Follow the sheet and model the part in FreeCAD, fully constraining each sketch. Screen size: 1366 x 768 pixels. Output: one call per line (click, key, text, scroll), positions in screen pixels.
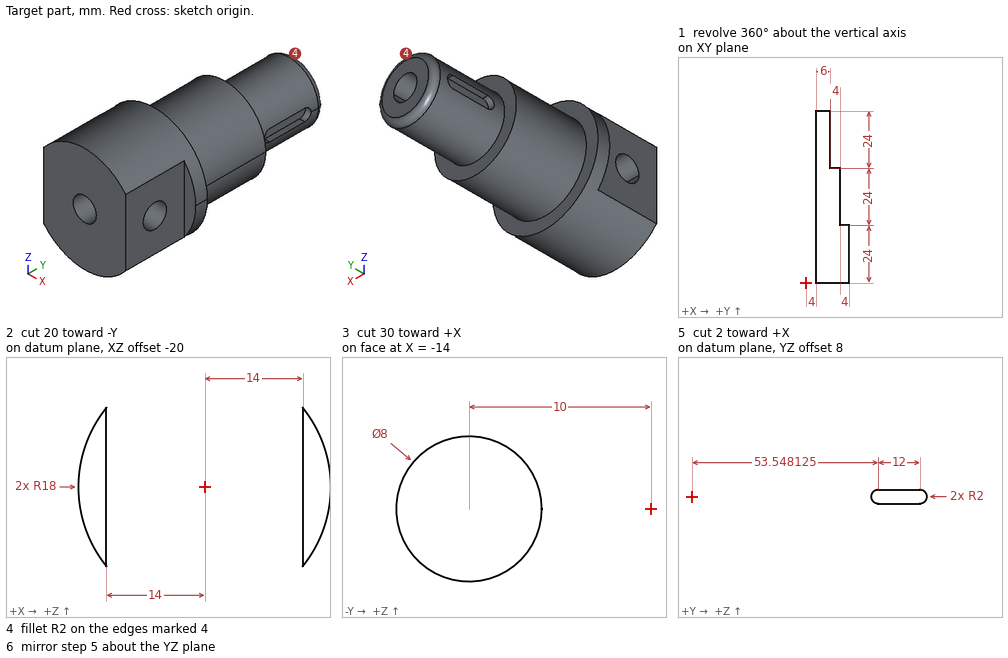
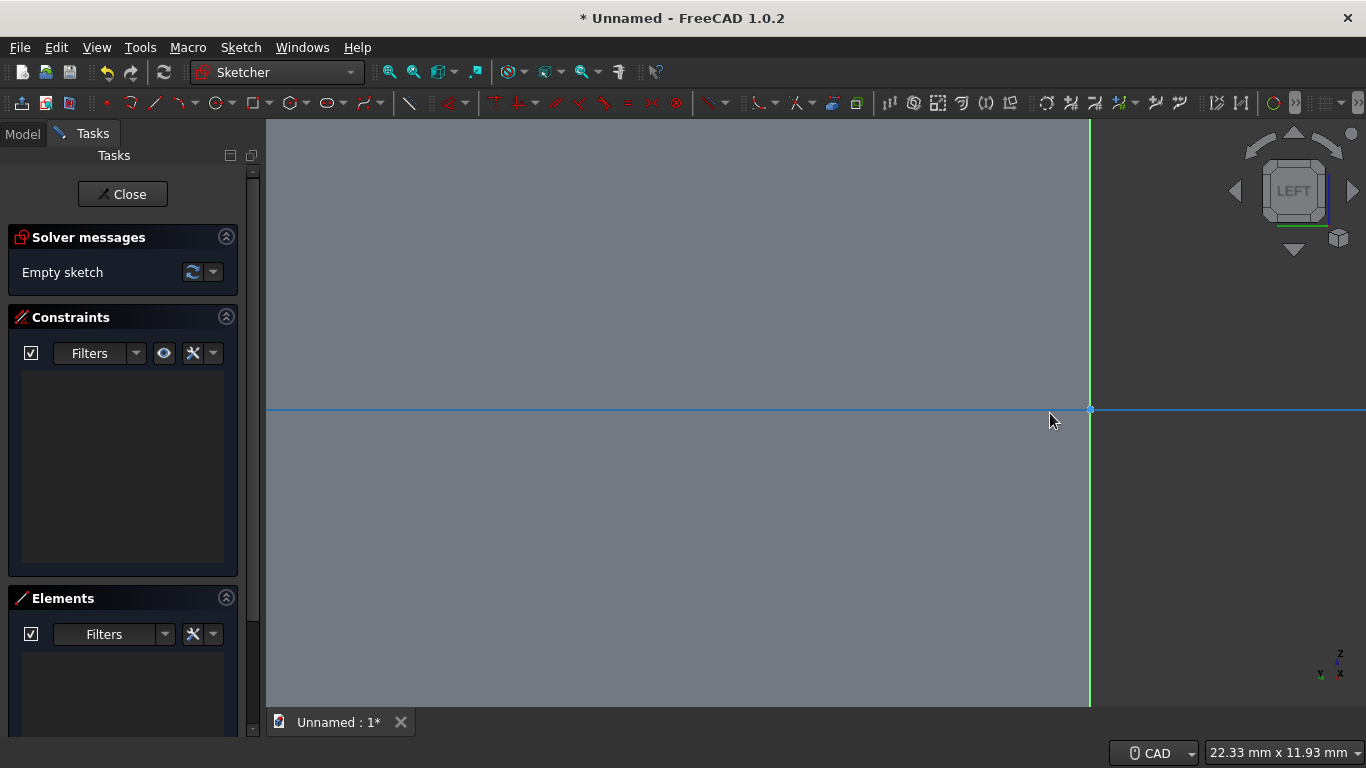
click(216, 104)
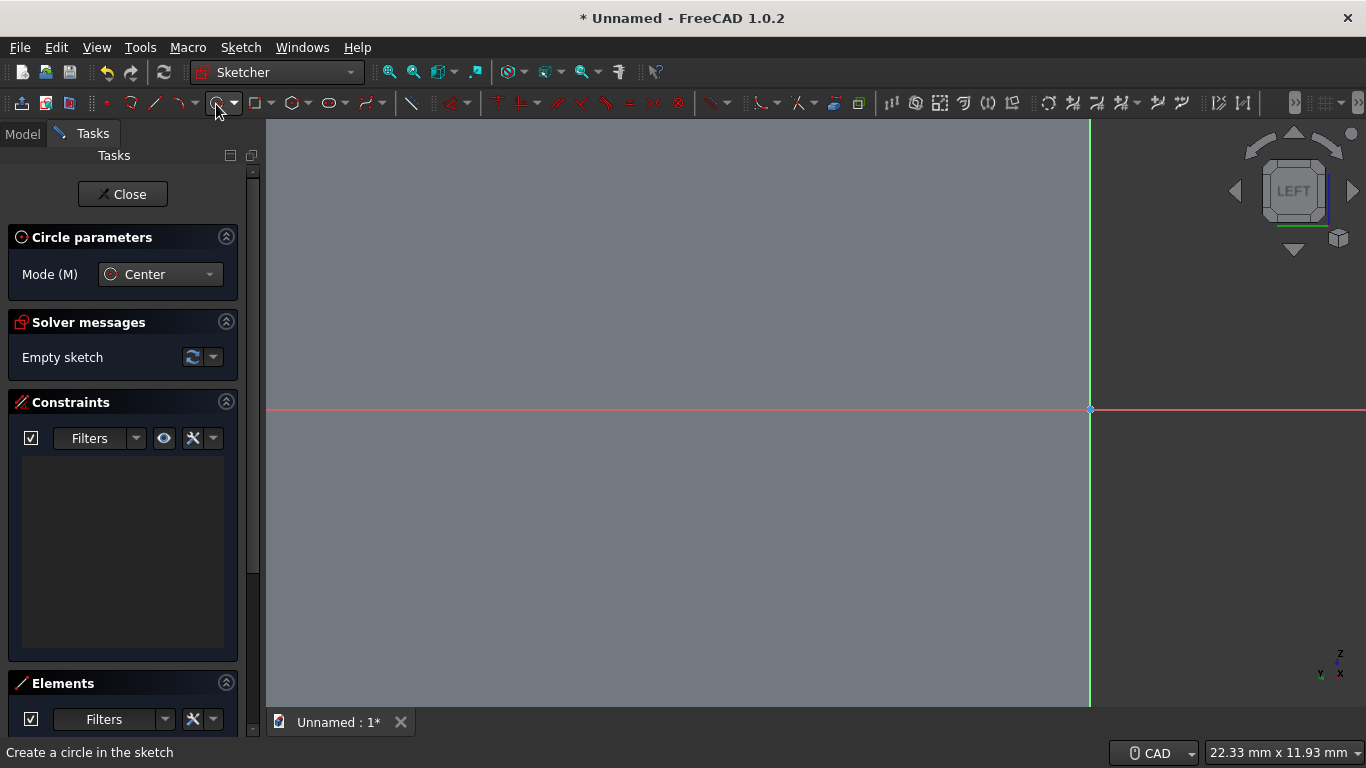
click(597, 410)
click(737, 270)
key(Escape)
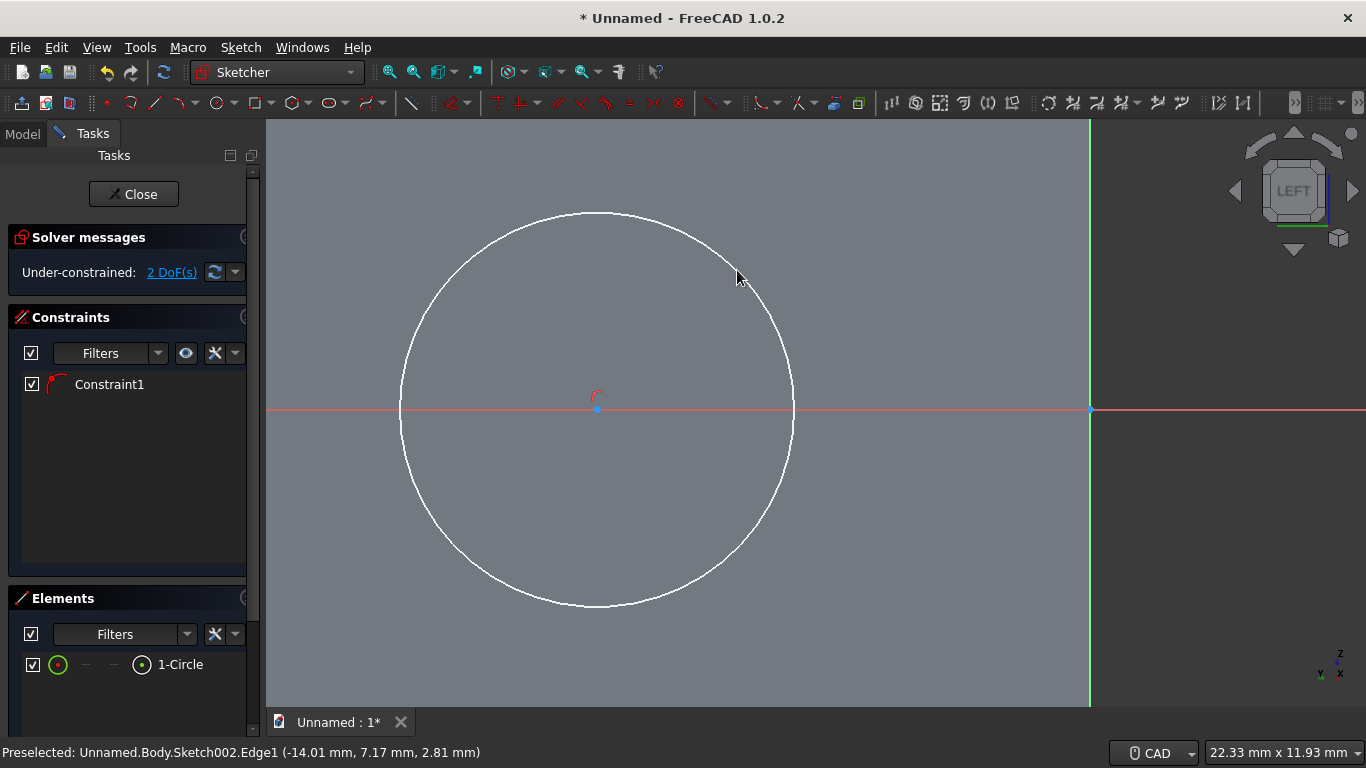
click(450, 104)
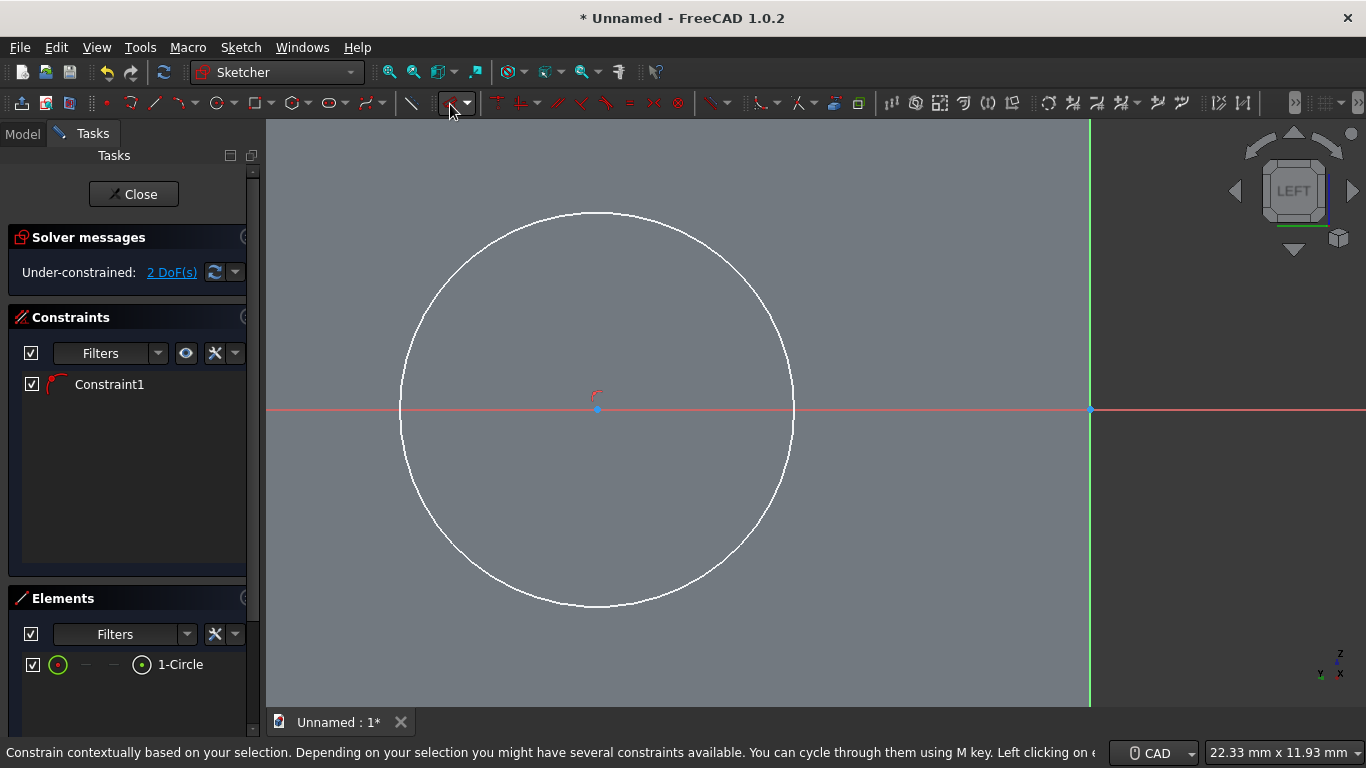
click(736, 270)
click(759, 247)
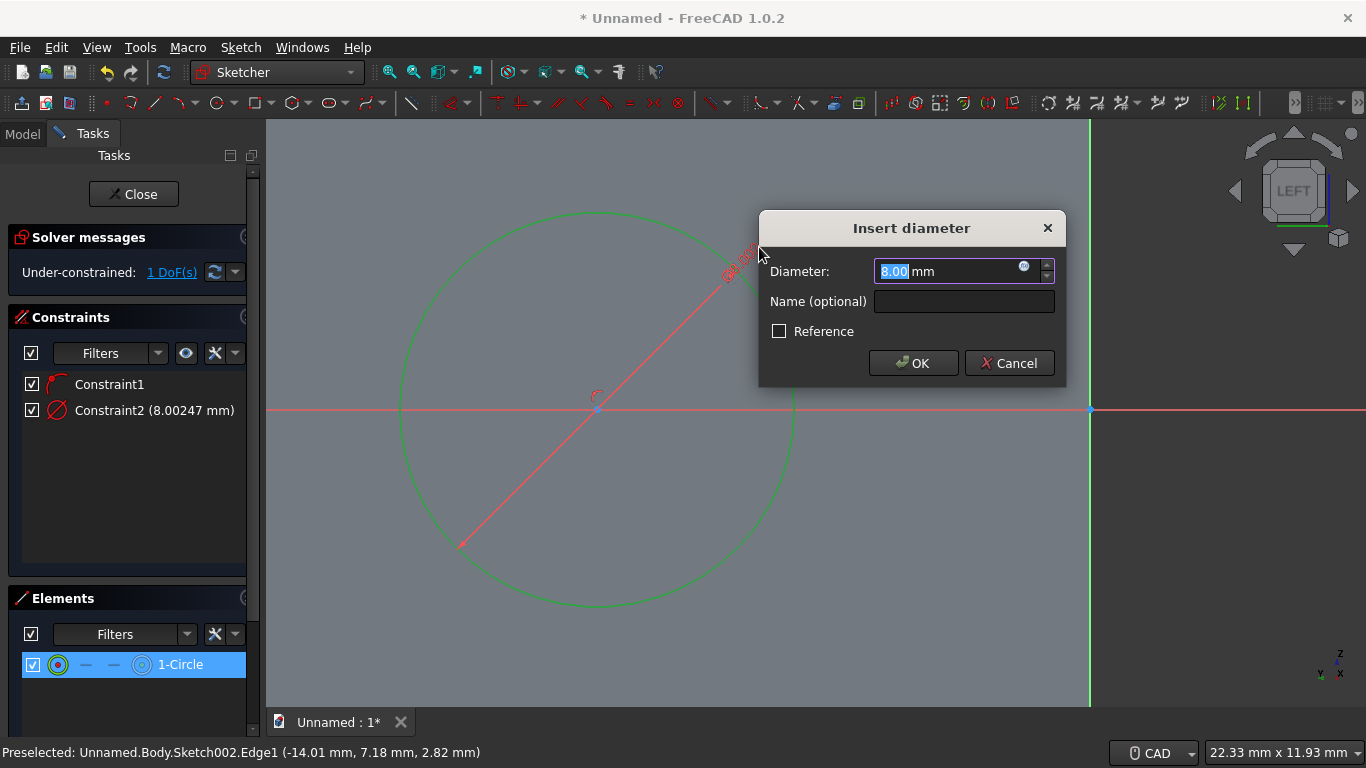
text(8)
key(Return)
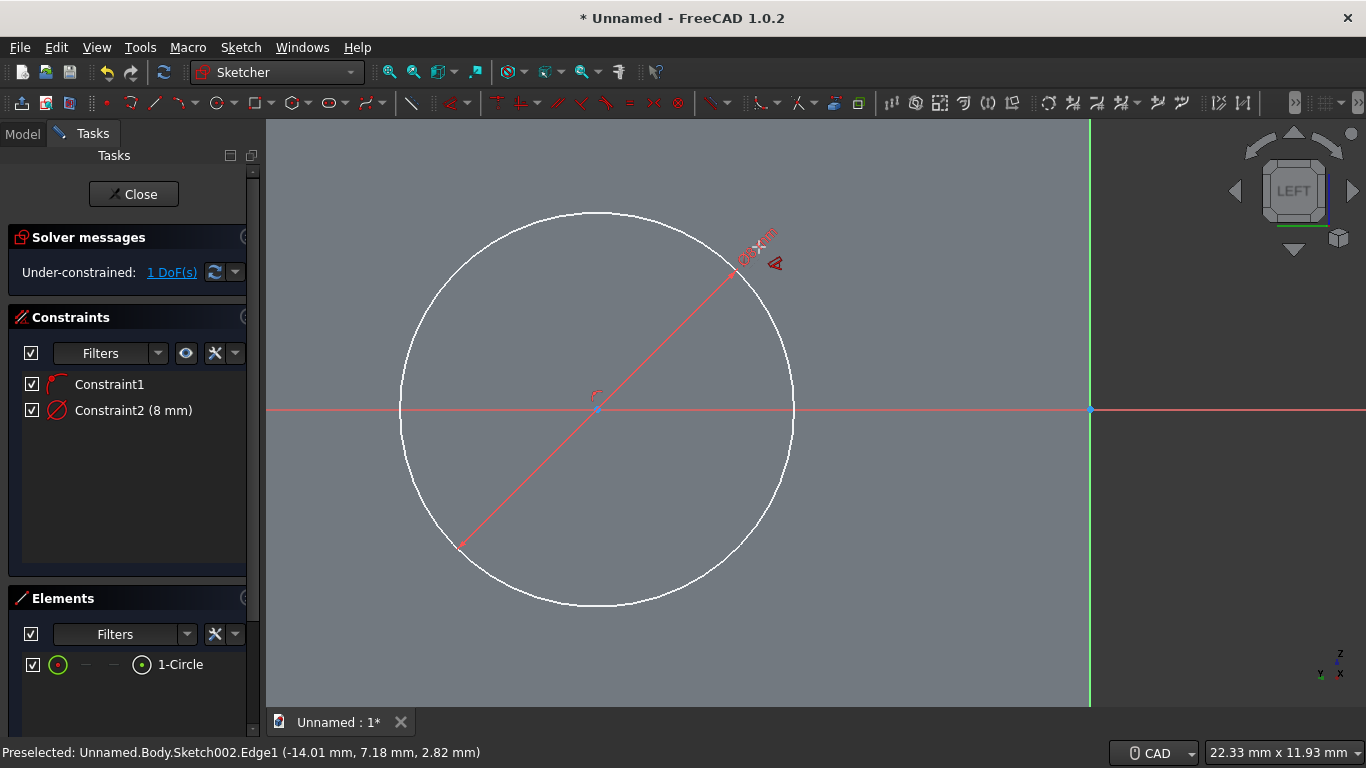
click(597, 410)
click(844, 444)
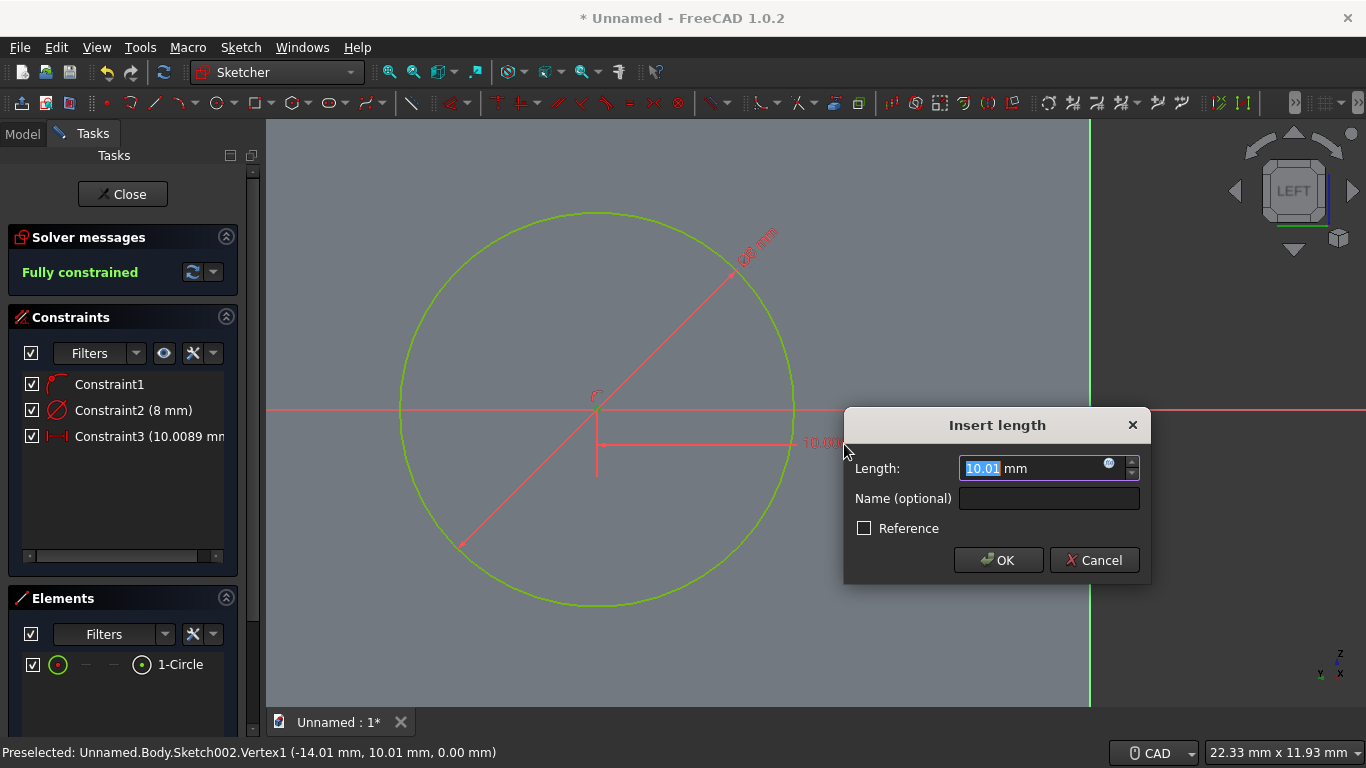
text(10)
key(Return)
key(Escape)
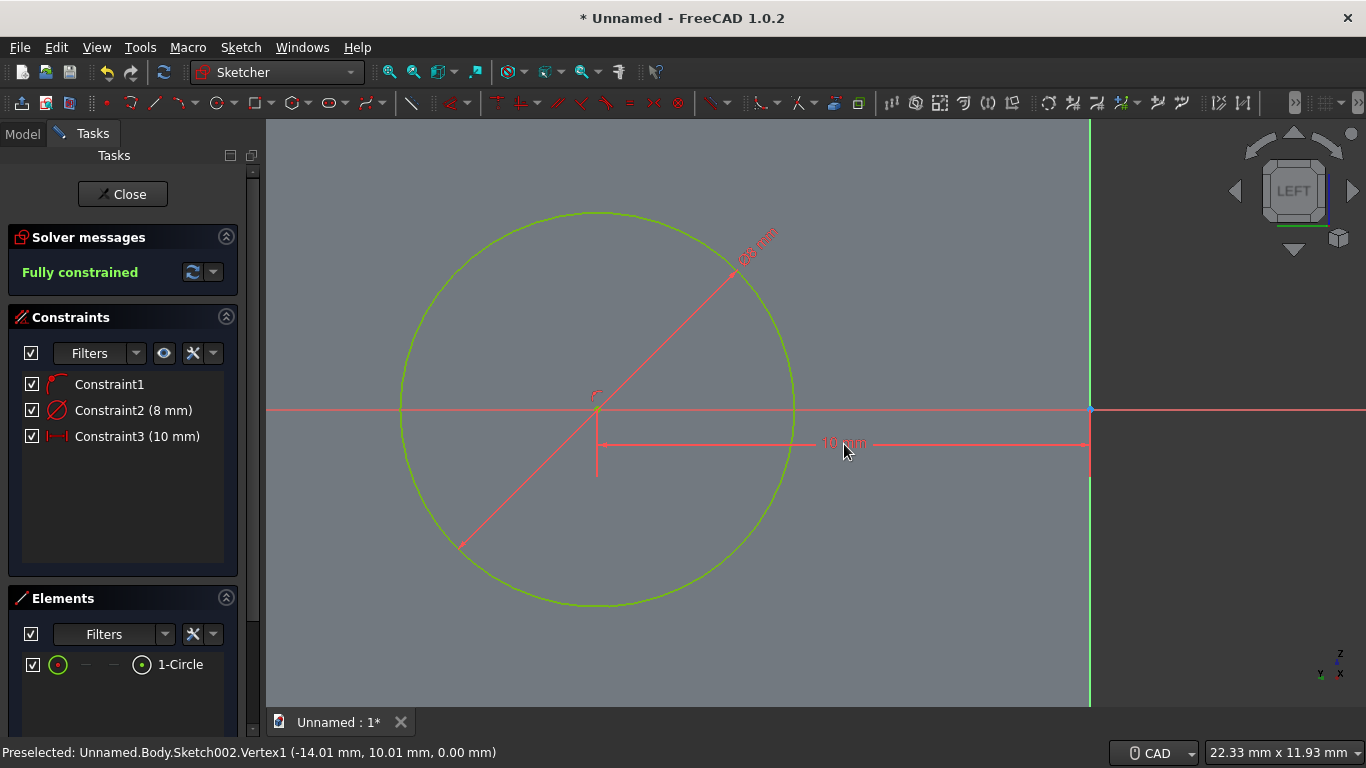
click(123, 194)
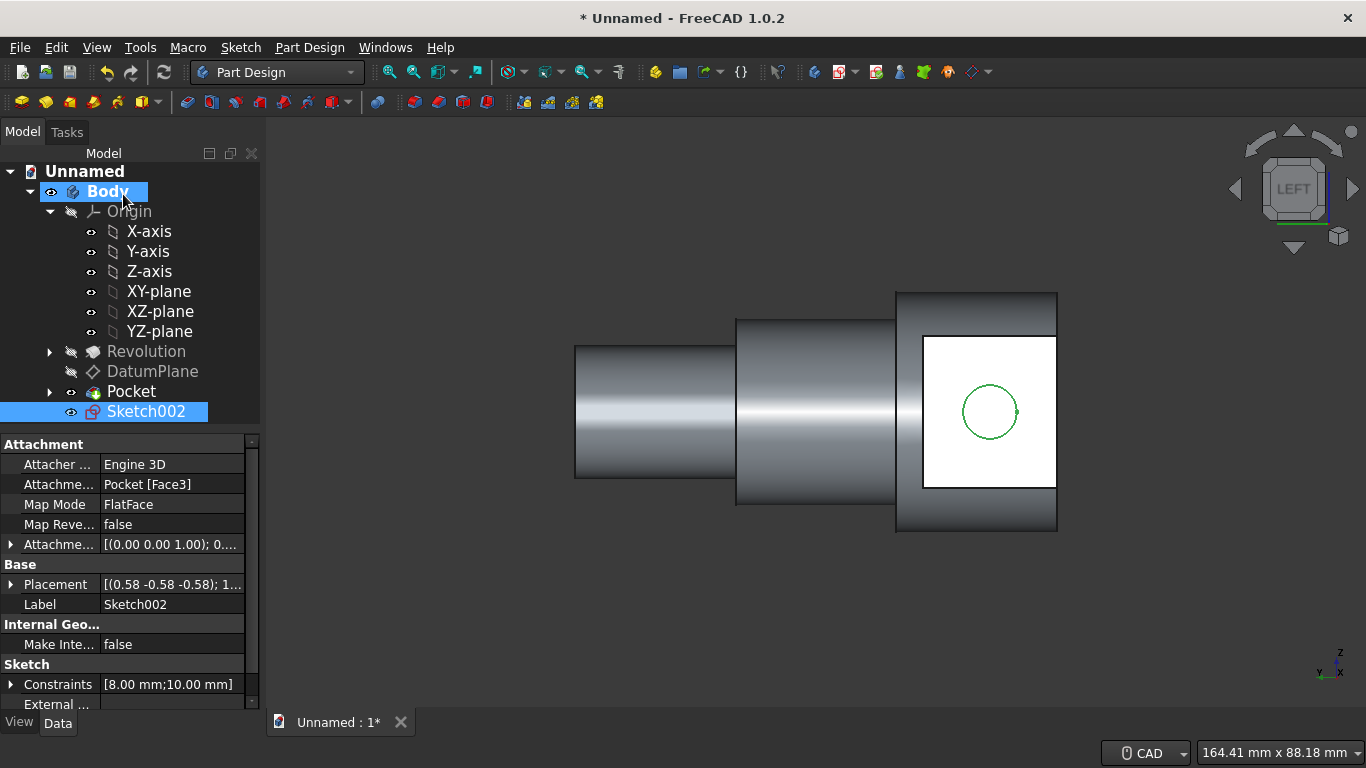
click(188, 102)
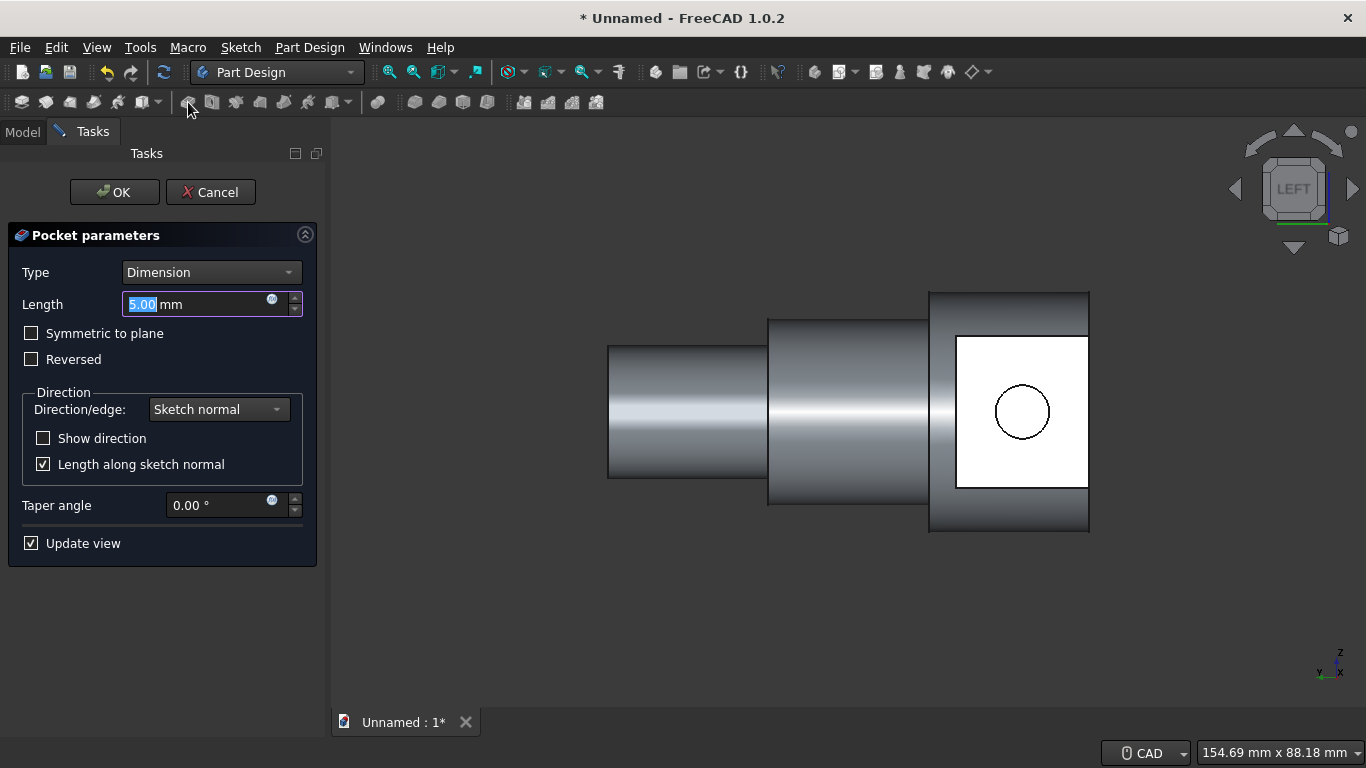
text(30)
key(Tab)